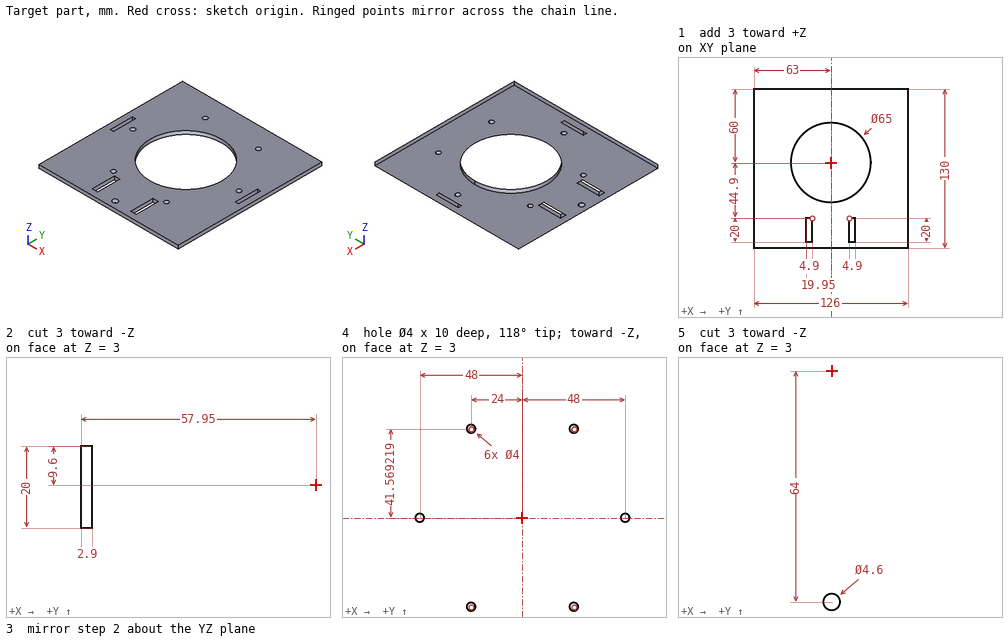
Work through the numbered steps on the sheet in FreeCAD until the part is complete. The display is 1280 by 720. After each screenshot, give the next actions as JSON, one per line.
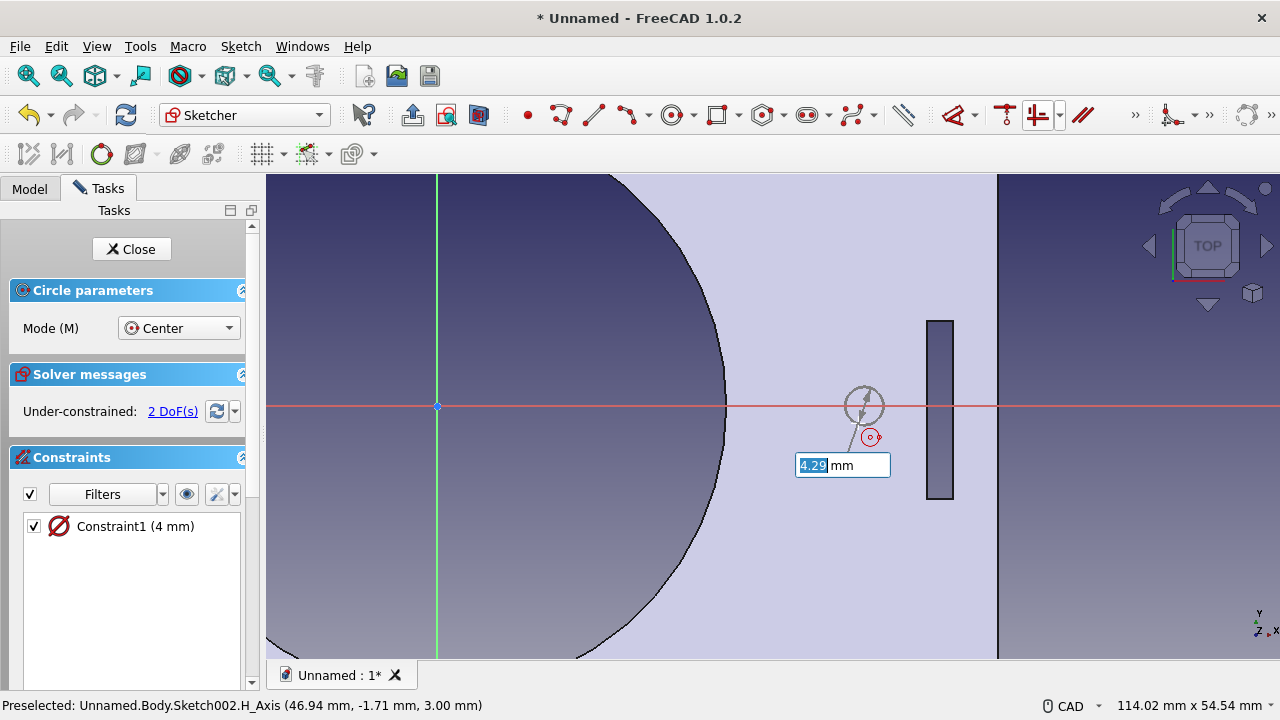
{"action": "type", "text": "4"}
{"action": "key", "text": "Return"}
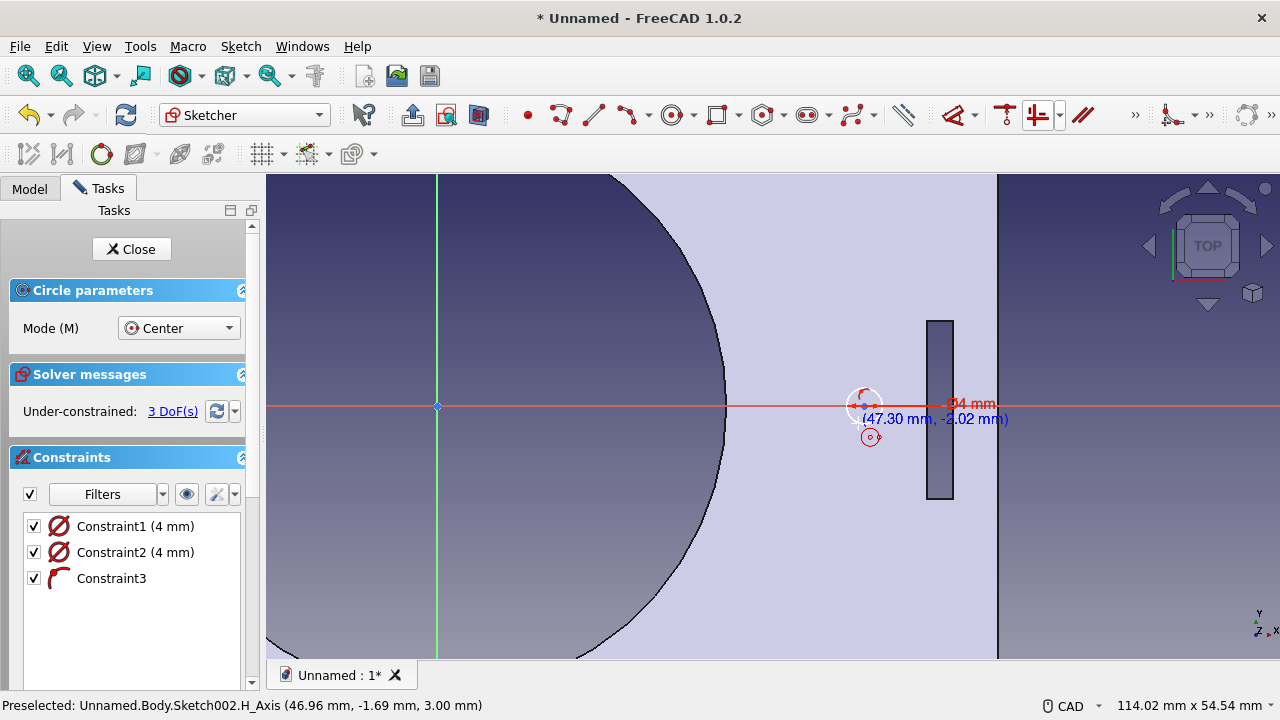
{"action": "scroll", "coordinate": [860, 423], "scroll_direction": "down", "scroll_amount": 5}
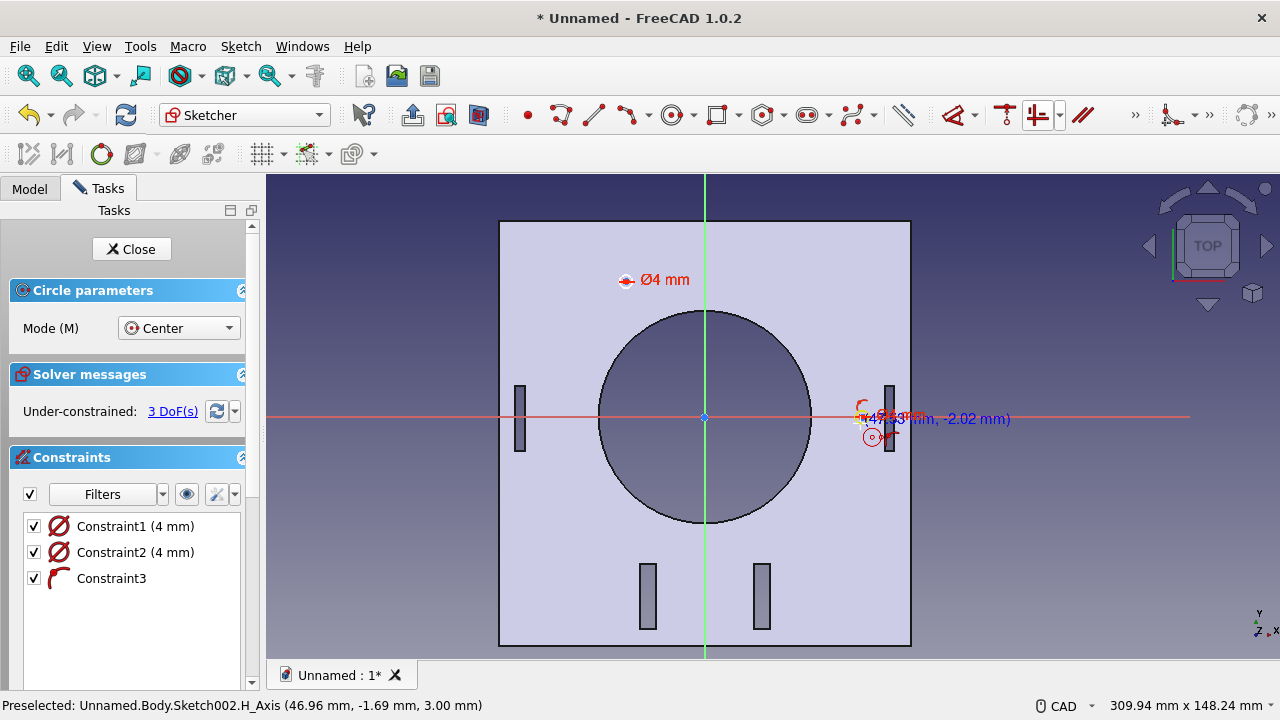
{"action": "scroll", "coordinate": [783, 281], "scroll_direction": "up", "scroll_amount": 7}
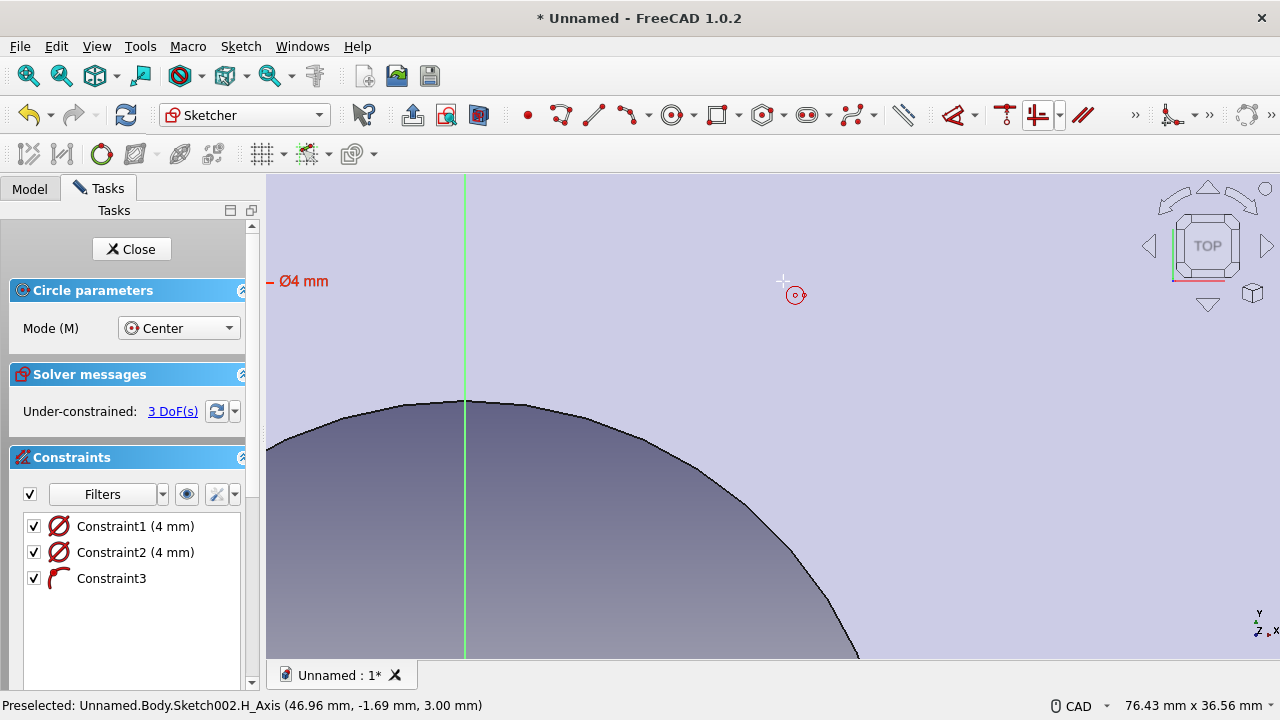
{"action": "scroll", "coordinate": [783, 280], "scroll_direction": "down", "scroll_amount": 7}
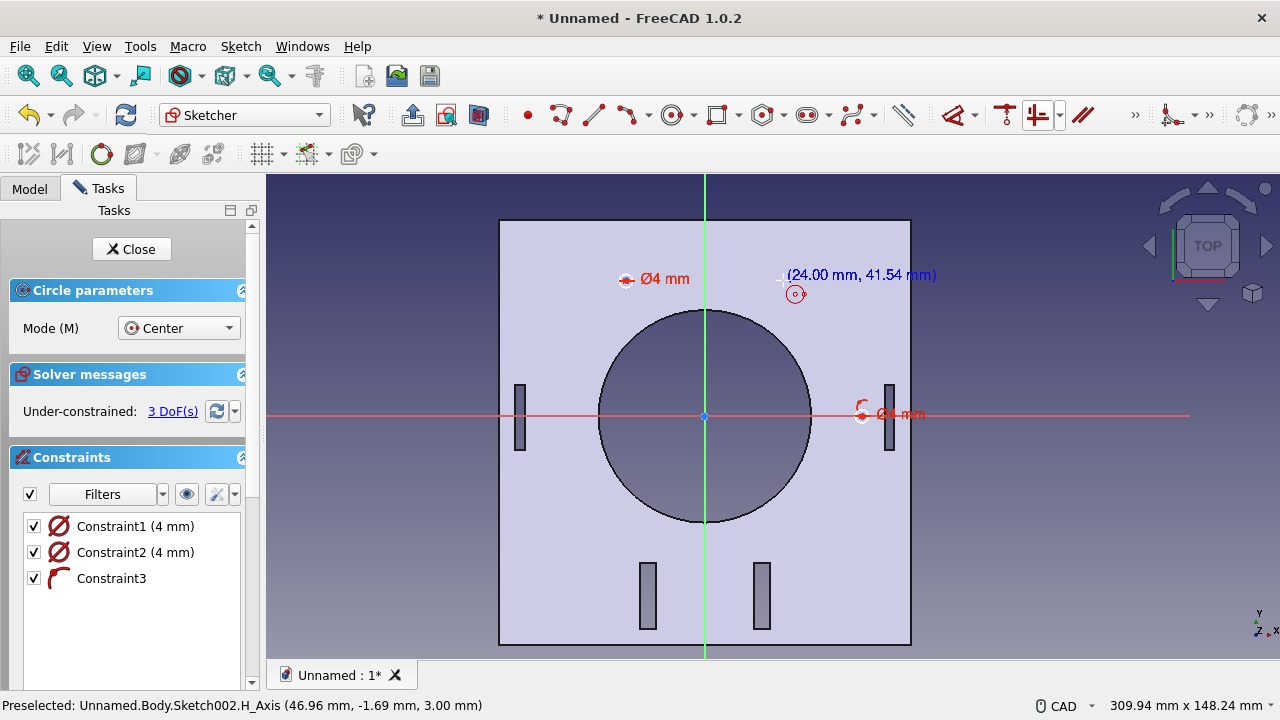
{"action": "left_click", "coordinate": [783, 280]}
{"action": "mouse_move", "coordinate": [788, 276]}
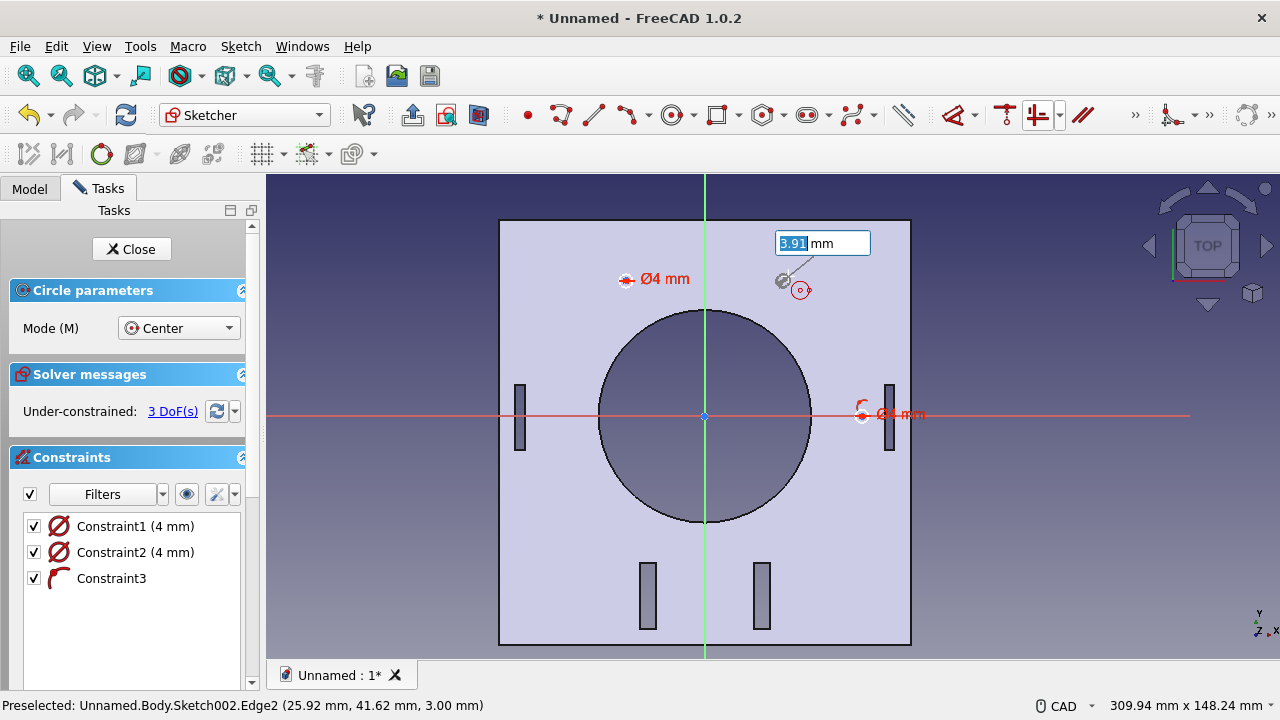
{"action": "type", "text": "4"}
{"action": "key", "text": "Return"}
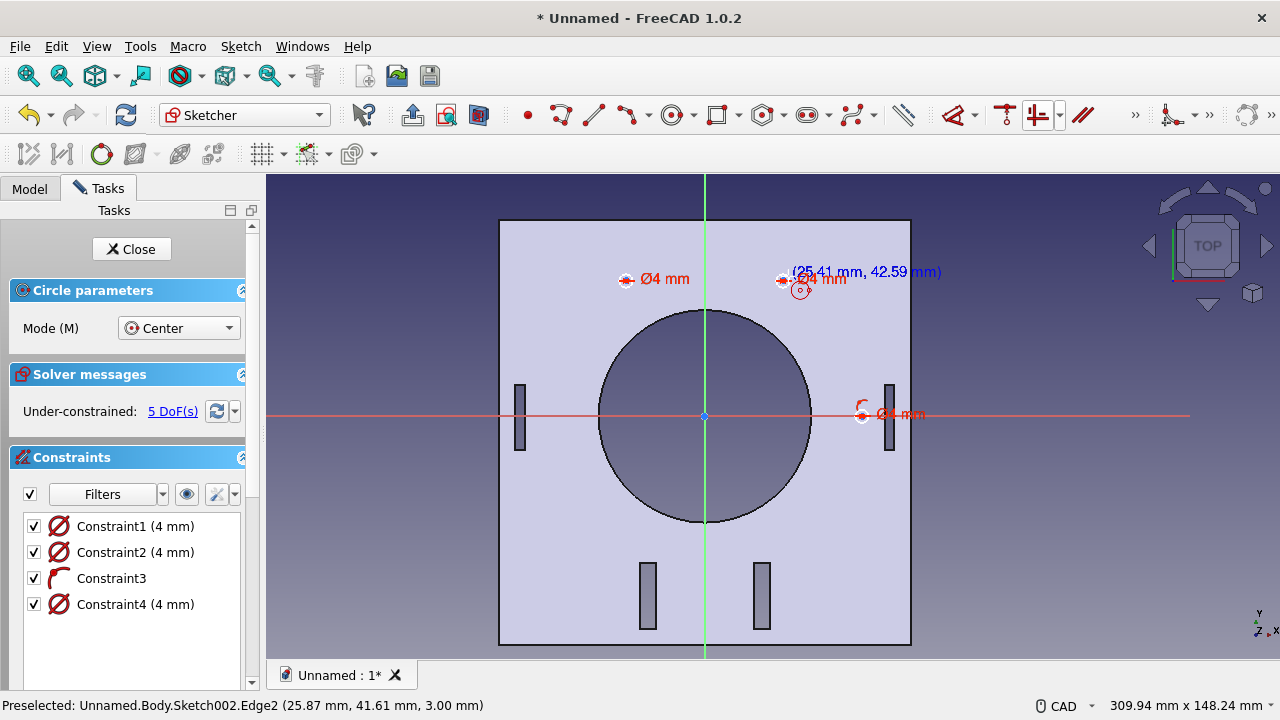
{"action": "scroll", "coordinate": [783, 552], "scroll_direction": "up", "scroll_amount": 7}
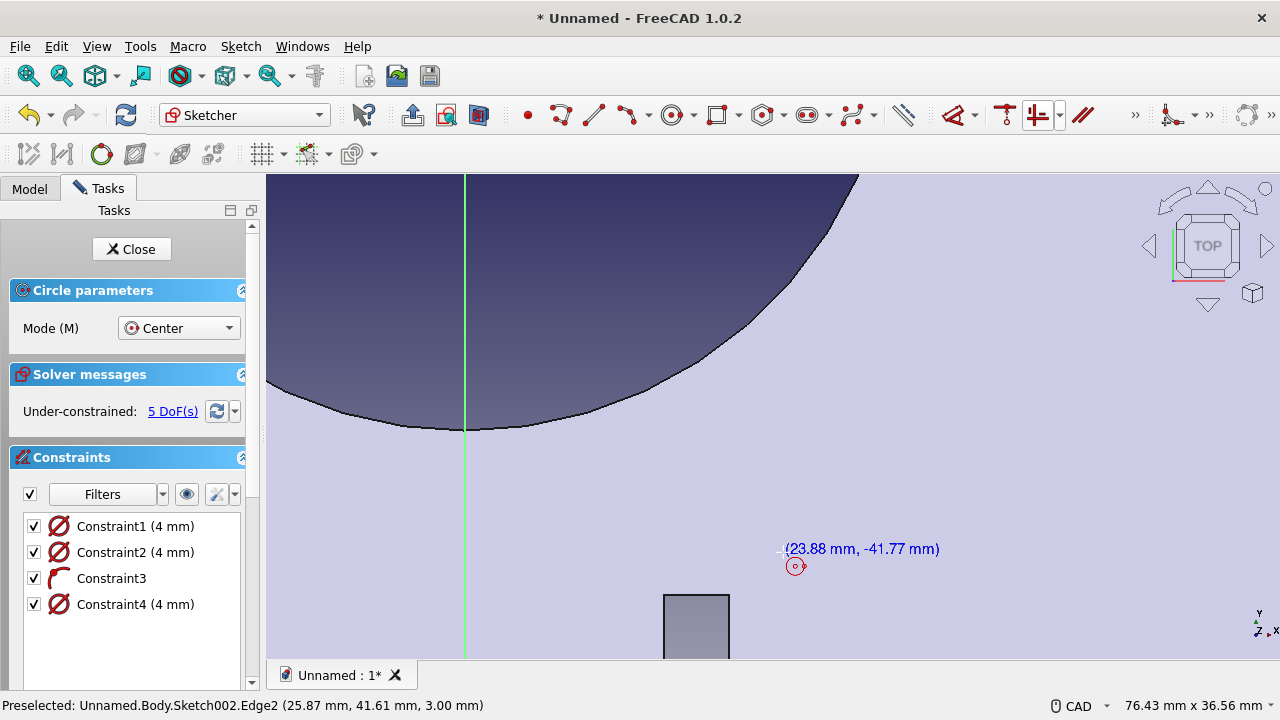
{"action": "scroll", "coordinate": [783, 553], "scroll_direction": "down", "scroll_amount": 7}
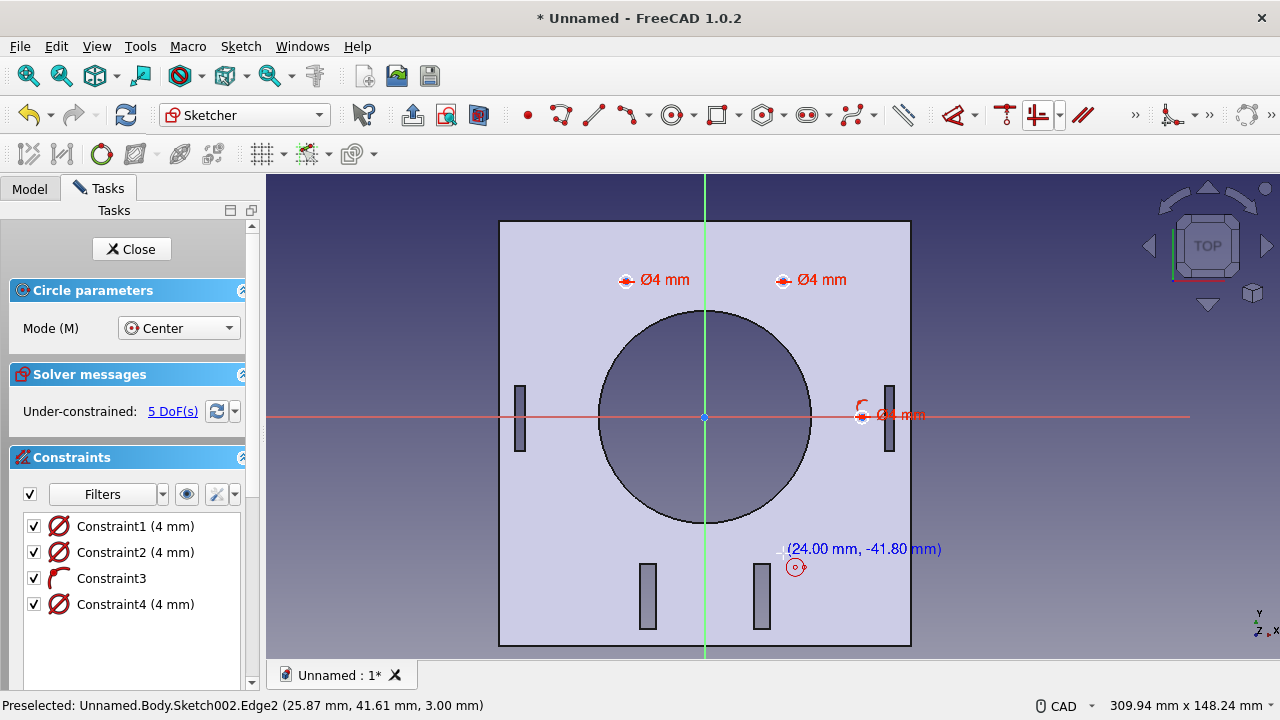
{"action": "left_click", "coordinate": [783, 553]}
{"action": "mouse_move", "coordinate": [788, 548]}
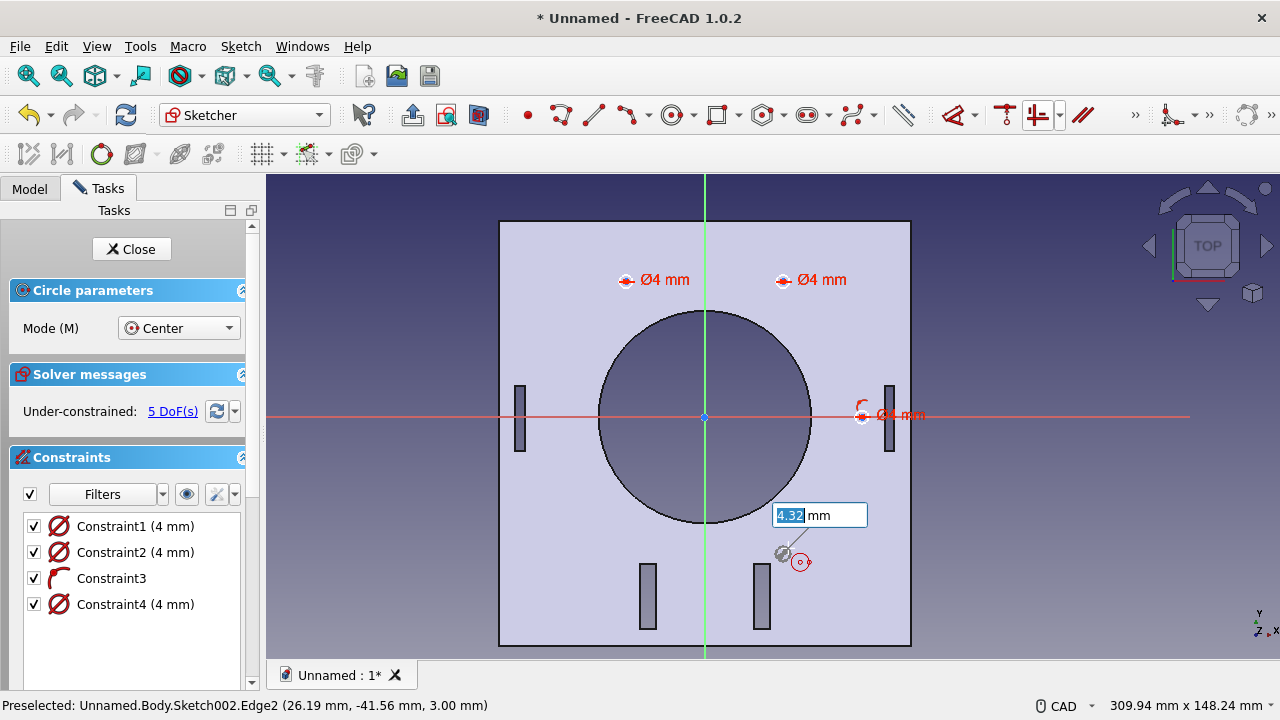
{"action": "type", "text": "4"}
{"action": "key", "text": "Return"}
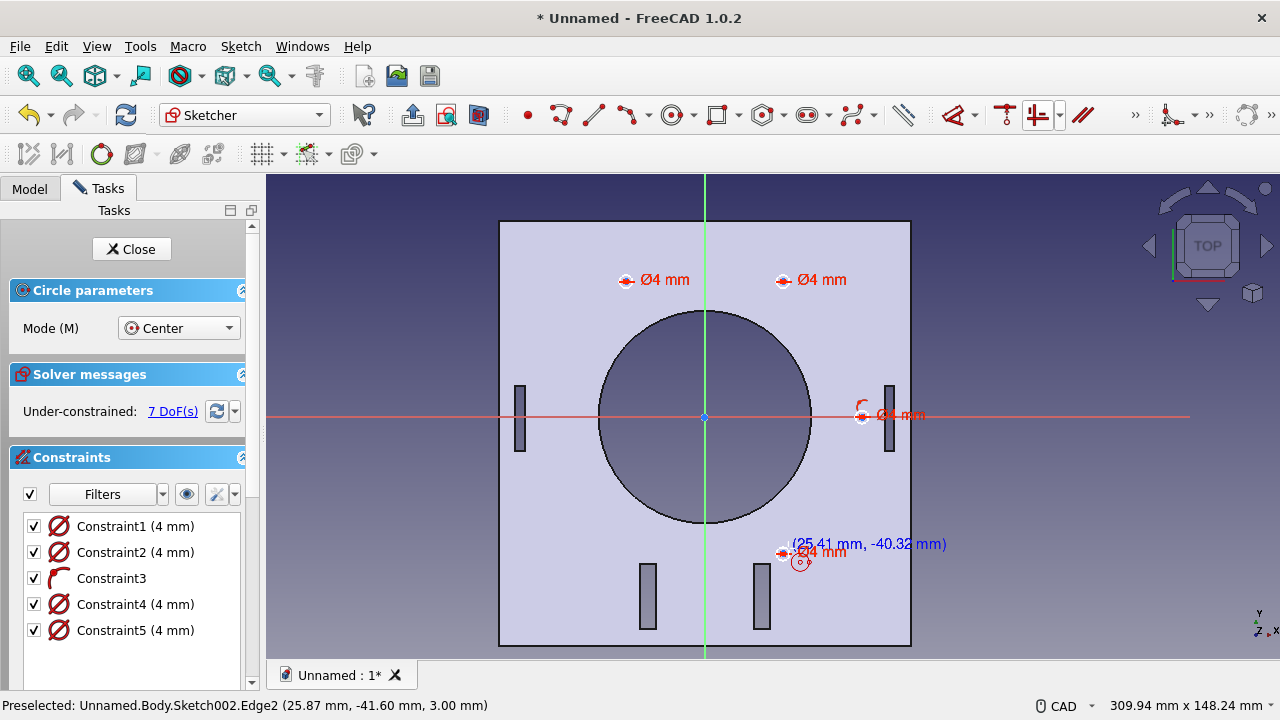
{"action": "scroll", "coordinate": [626, 553], "scroll_direction": "up", "scroll_amount": 7}